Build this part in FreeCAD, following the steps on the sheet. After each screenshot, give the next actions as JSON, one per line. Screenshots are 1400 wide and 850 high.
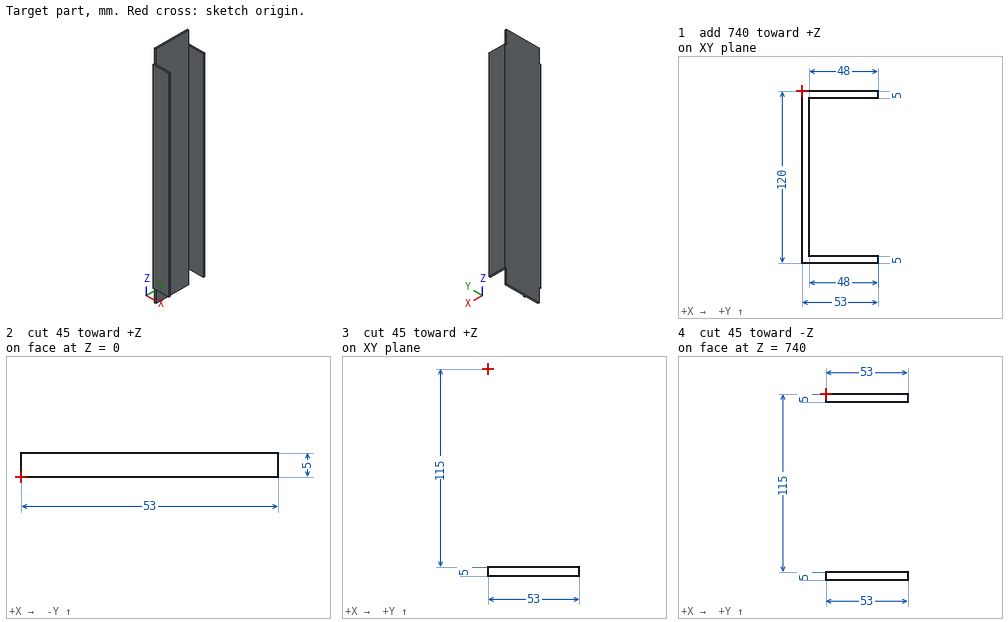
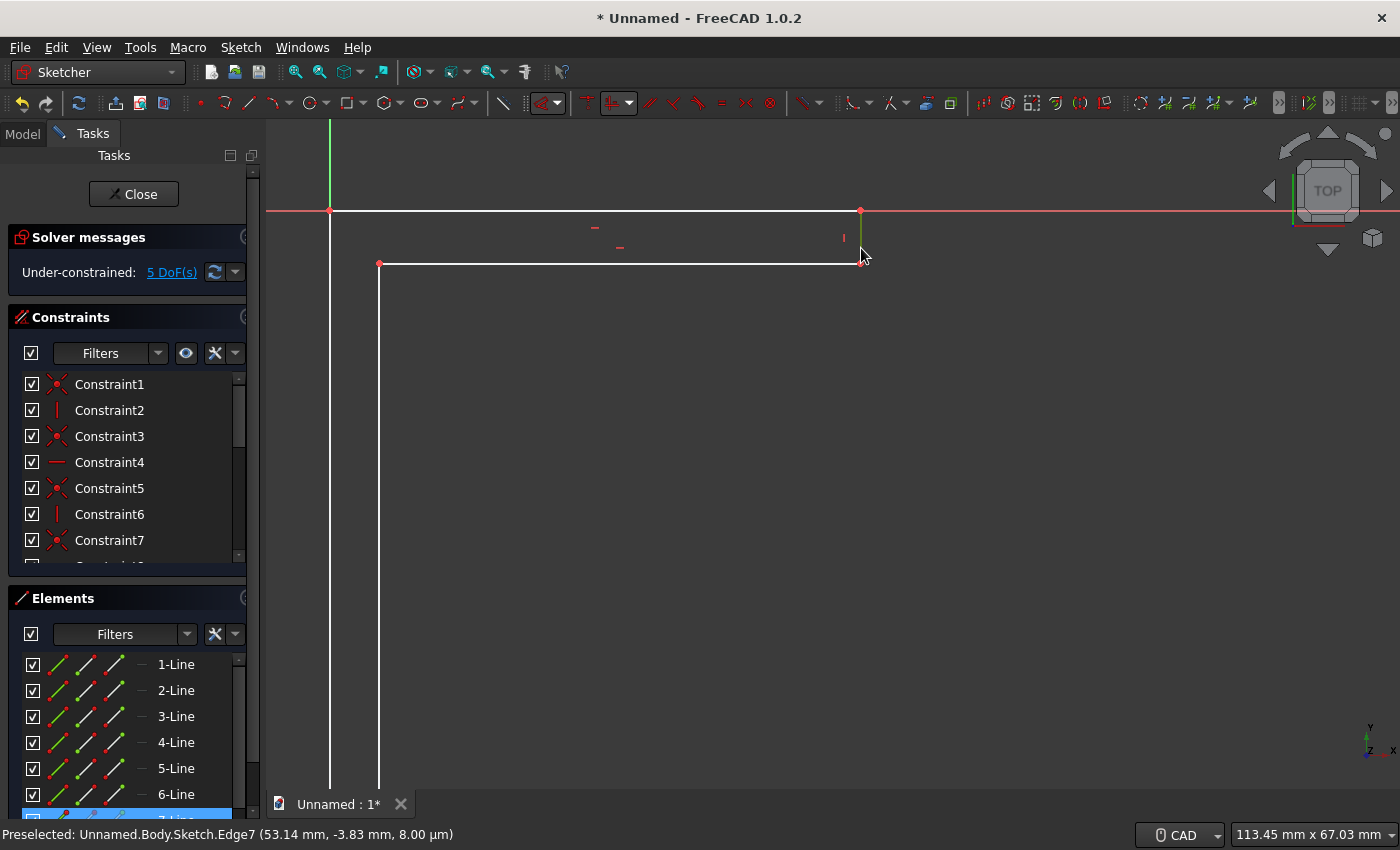
{"action": "key", "text": "i"}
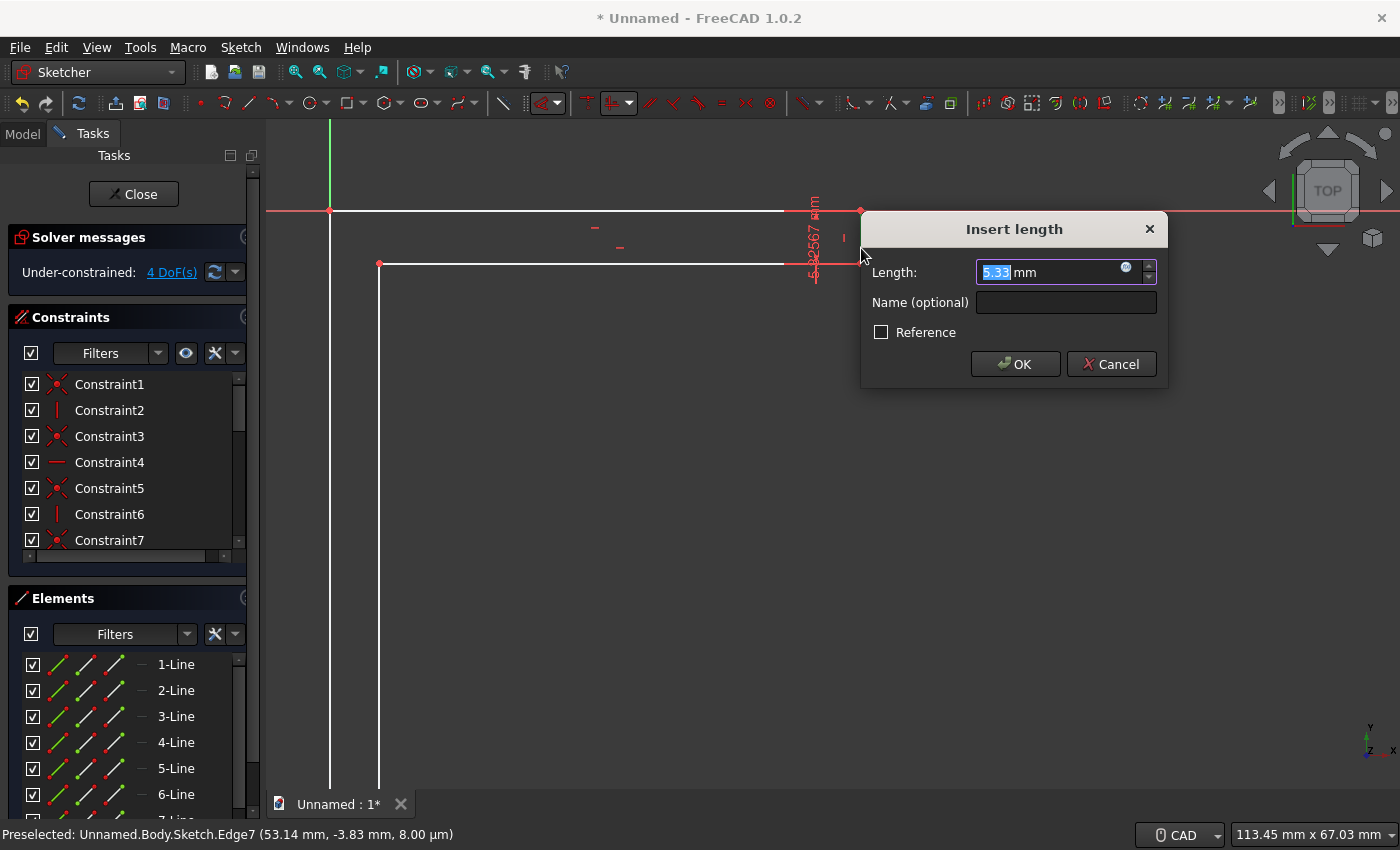
{"action": "type", "text": "5"}
{"action": "key", "text": "Return"}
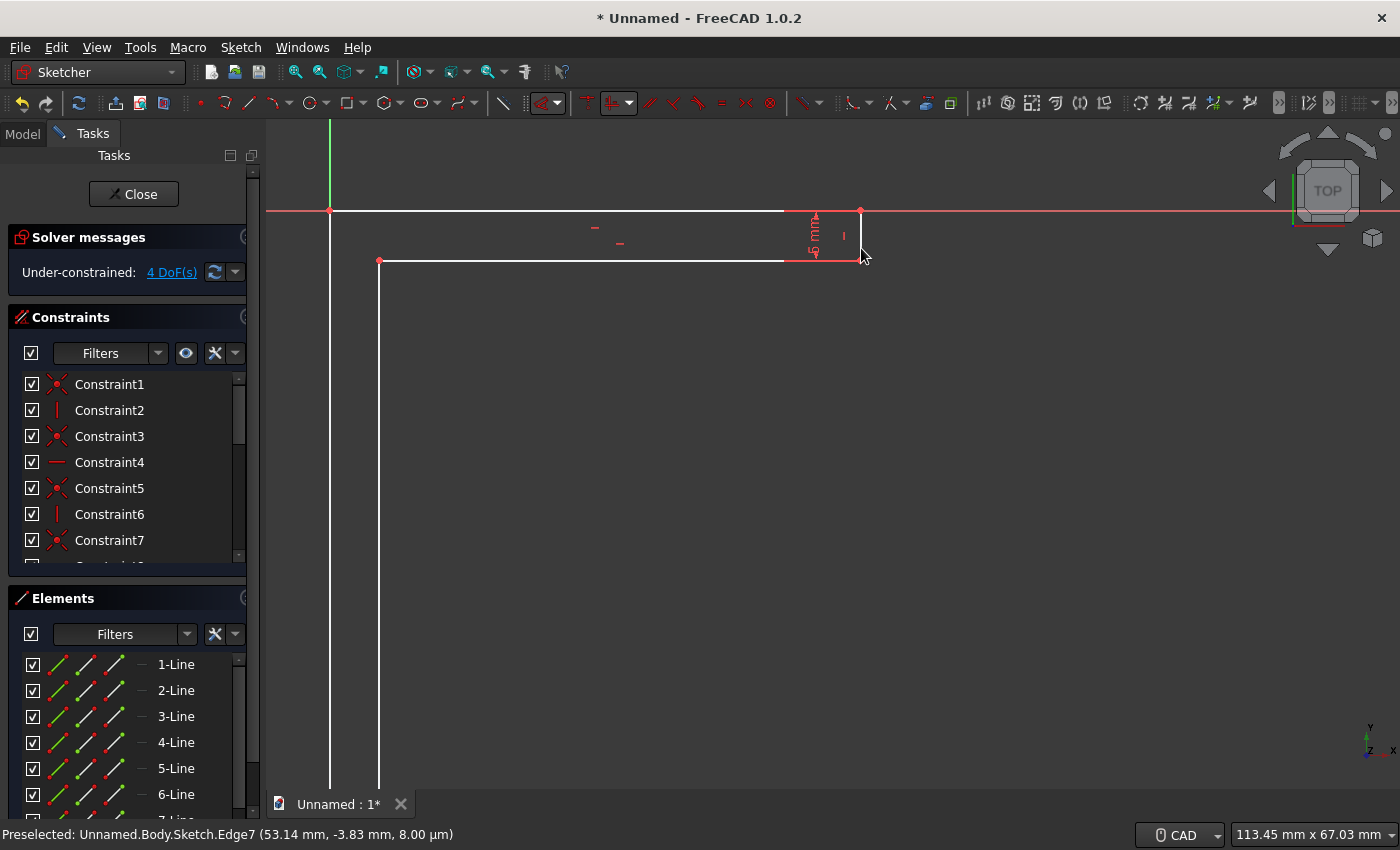
{"action": "scroll", "coordinate": [863, 247], "scroll_direction": "down", "scroll_amount": 5}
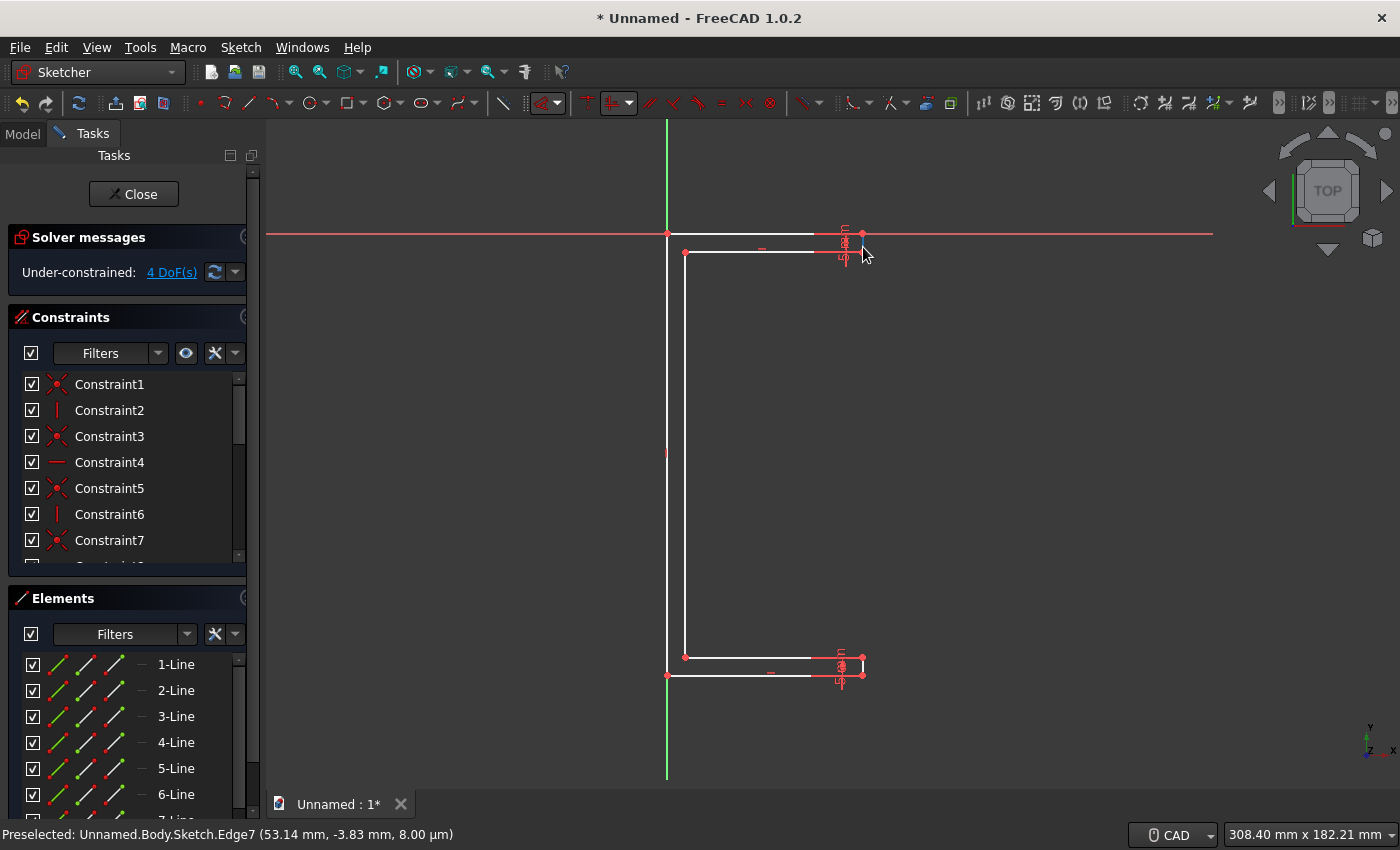
{"action": "left_click", "coordinate": [726, 676]}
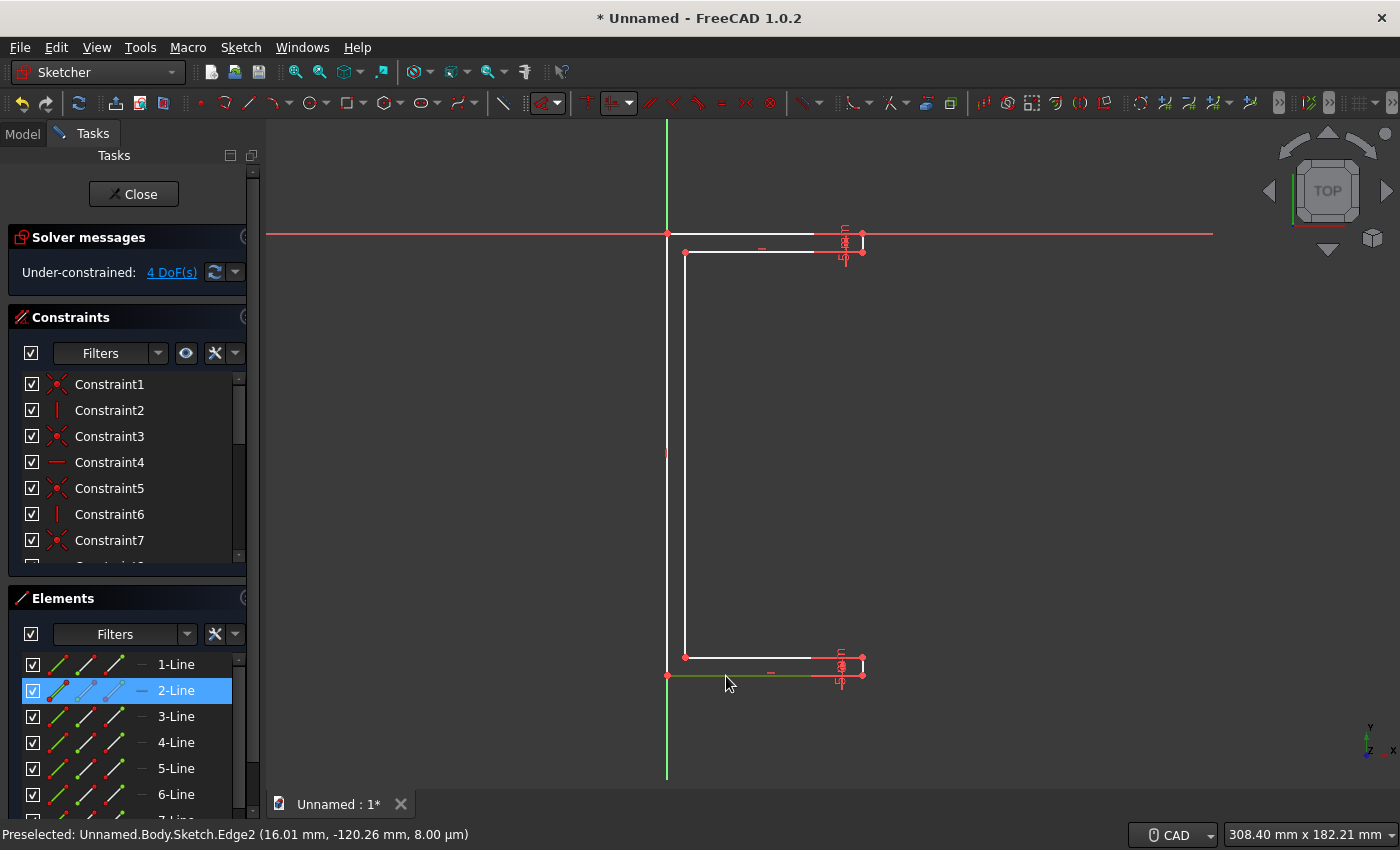
{"action": "left_click", "coordinate": [560, 104]}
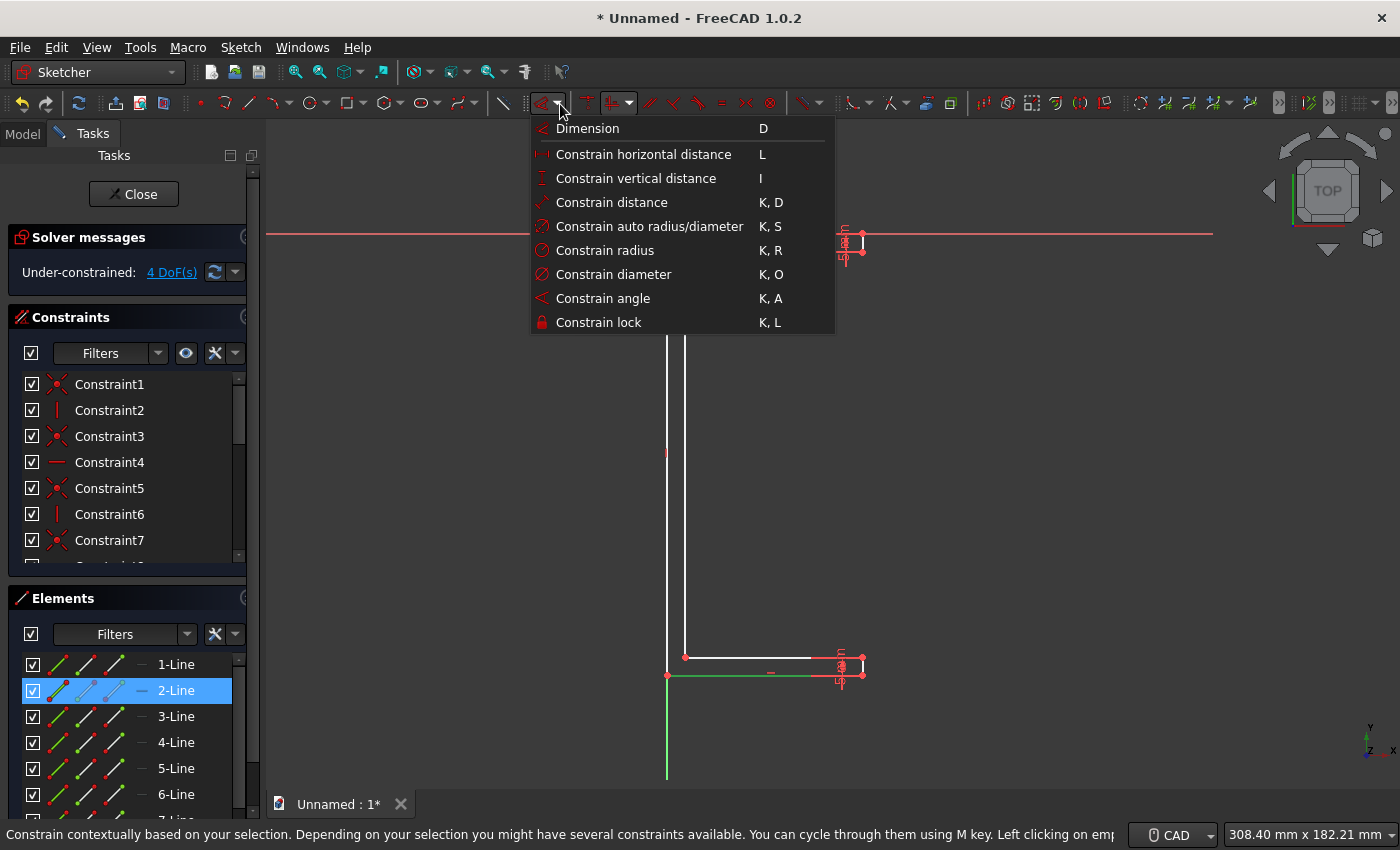
{"action": "left_click", "coordinate": [683, 154]}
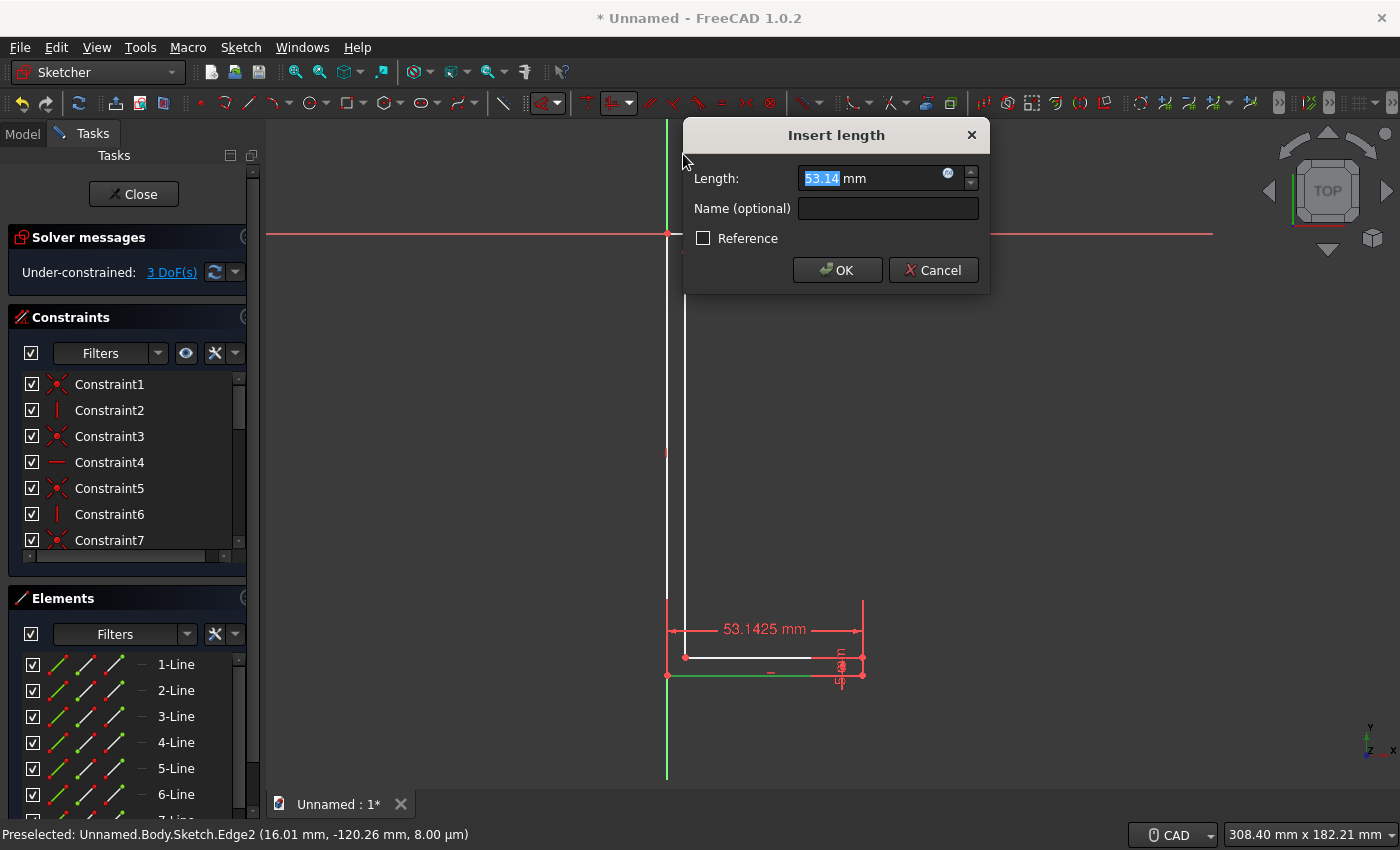
{"action": "type", "text": "53"}
{"action": "key", "text": "Return"}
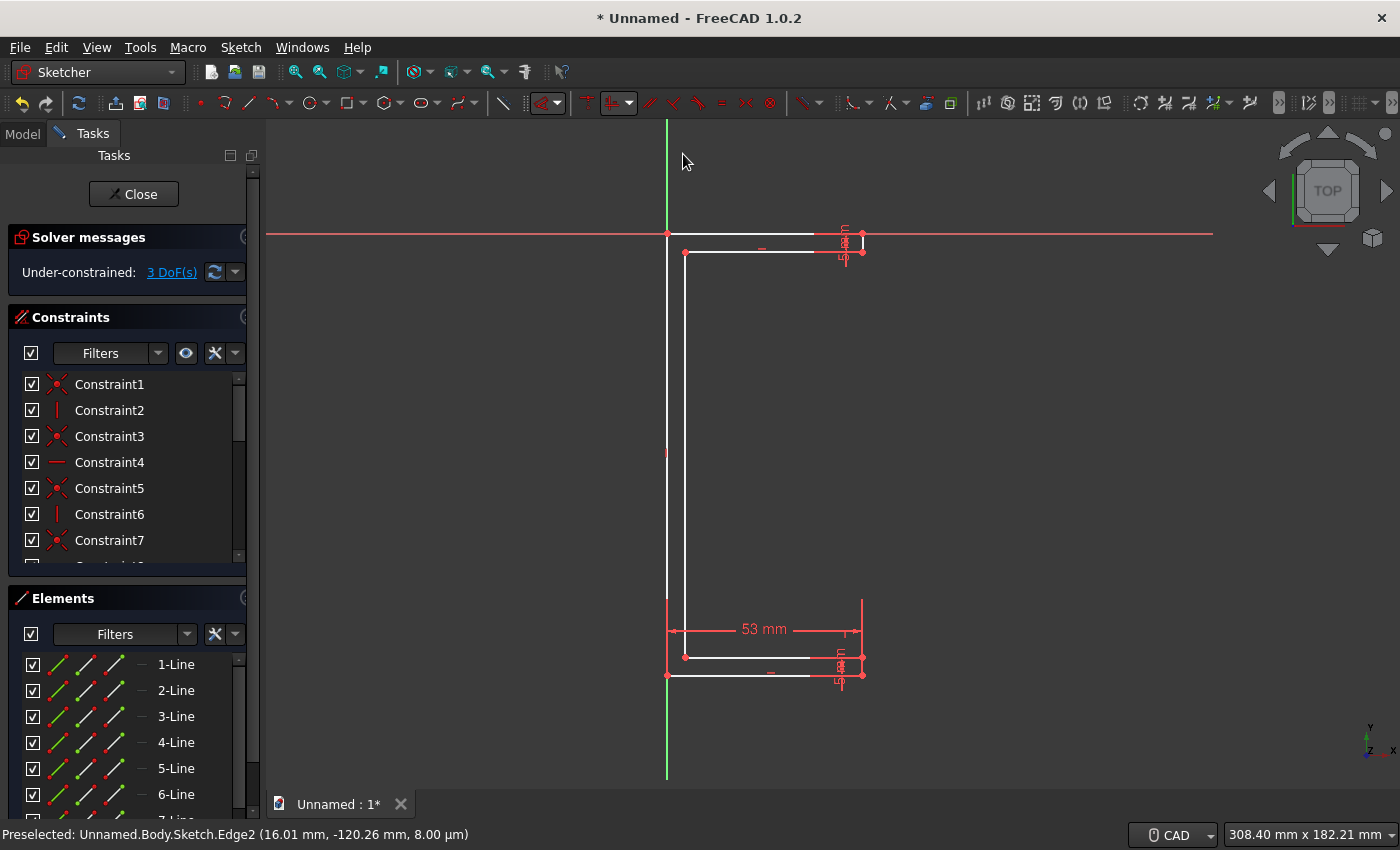
{"action": "left_click", "coordinate": [809, 658]}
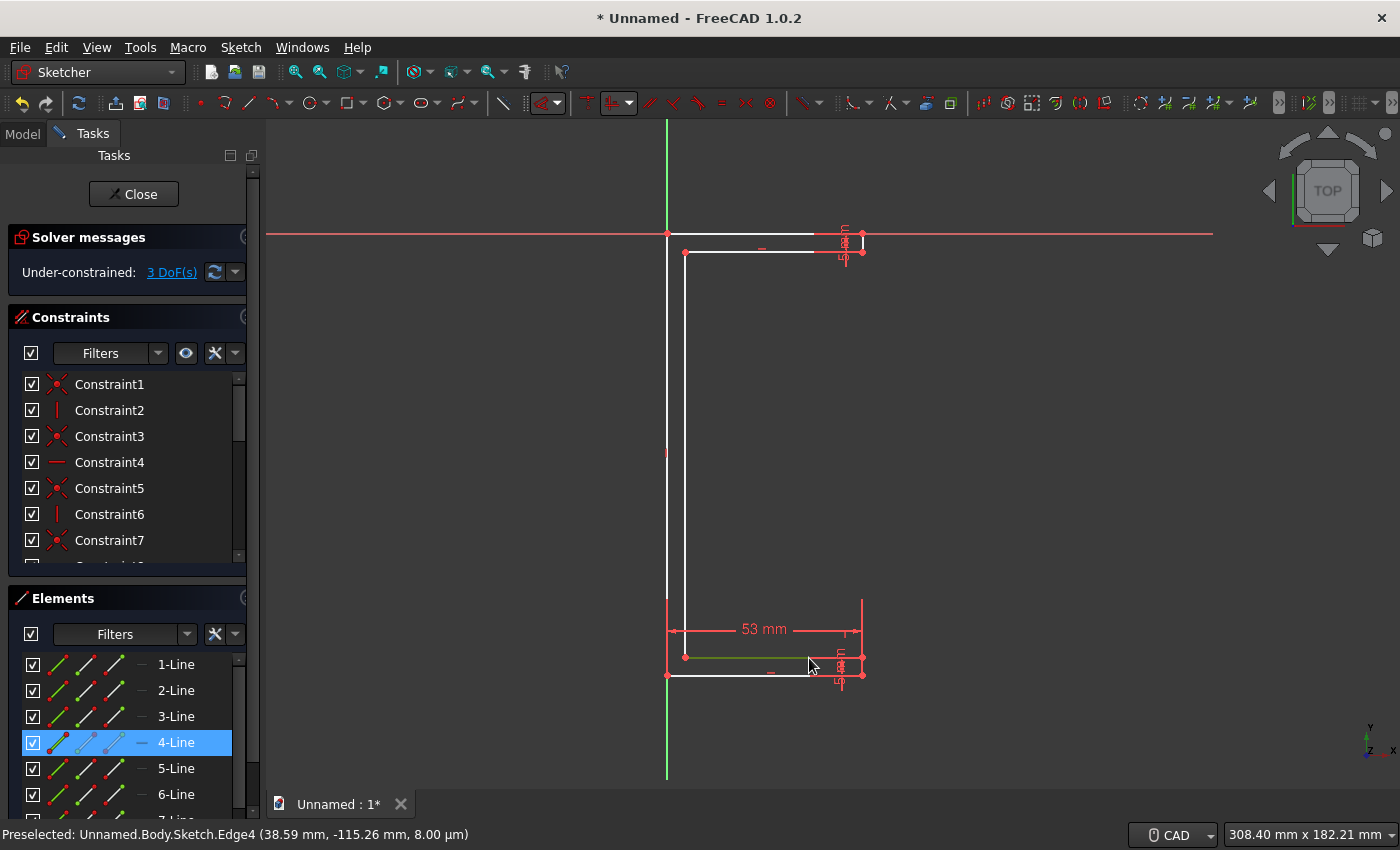
{"action": "key", "text": "l"}